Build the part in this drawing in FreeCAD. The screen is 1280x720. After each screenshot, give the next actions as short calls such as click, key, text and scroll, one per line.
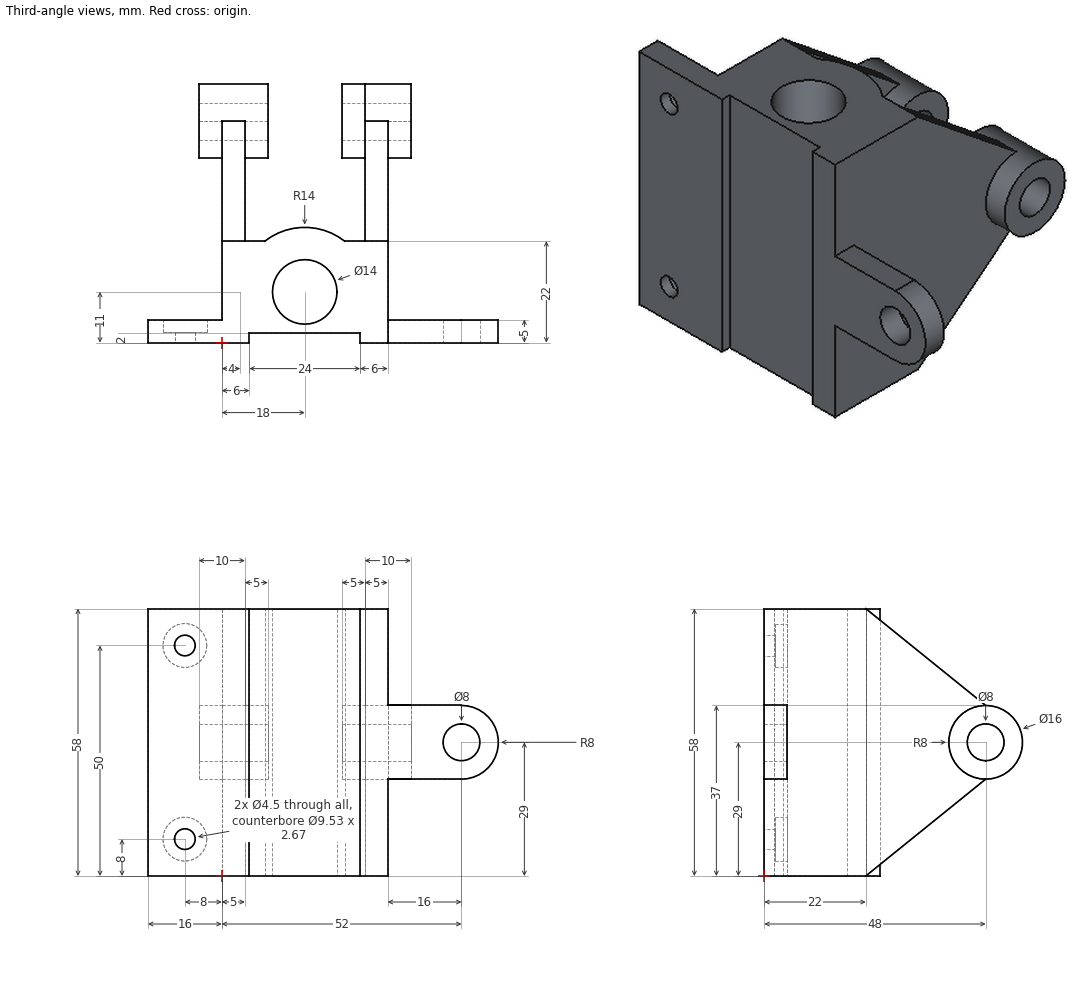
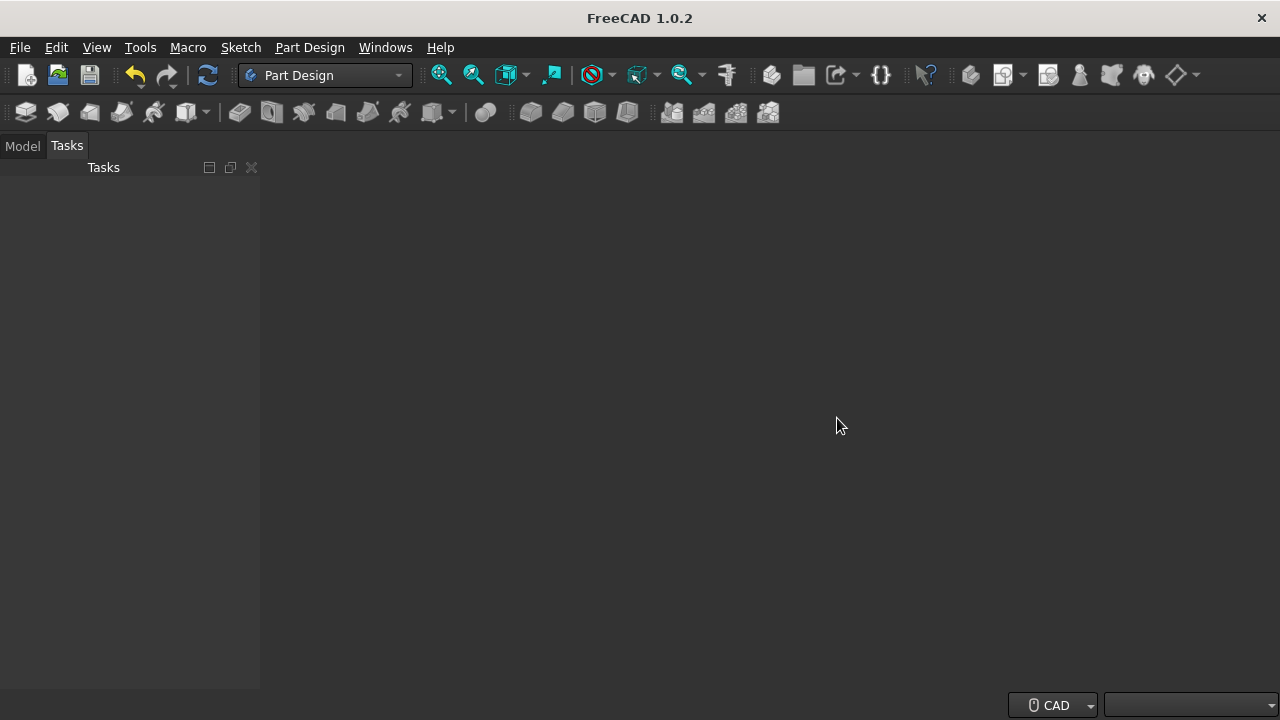
key(ctrl+n)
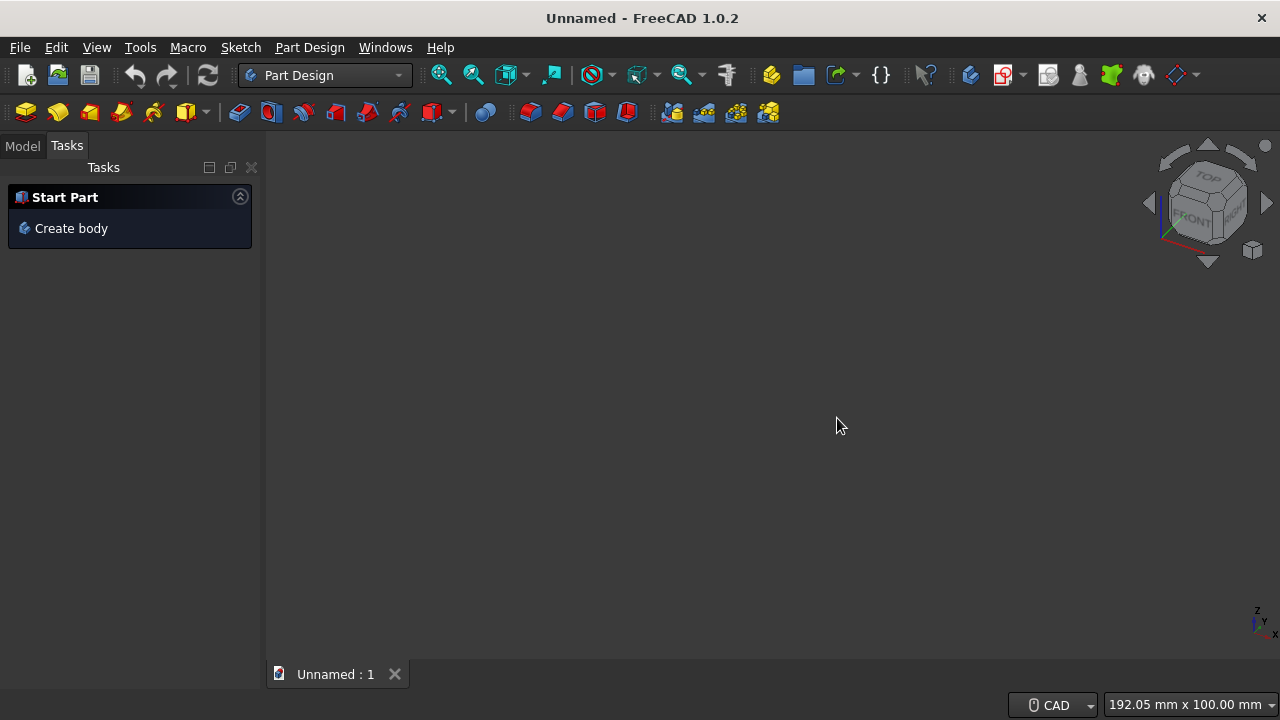
click(1004, 76)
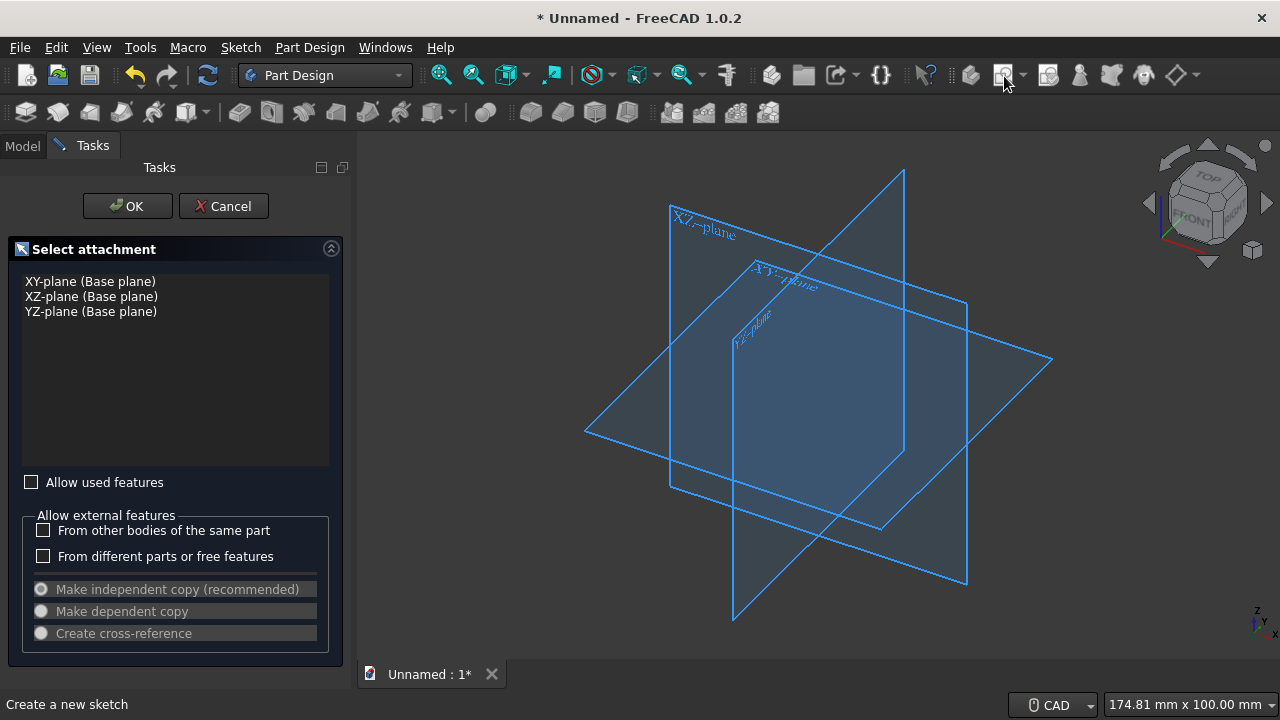
click(82, 282)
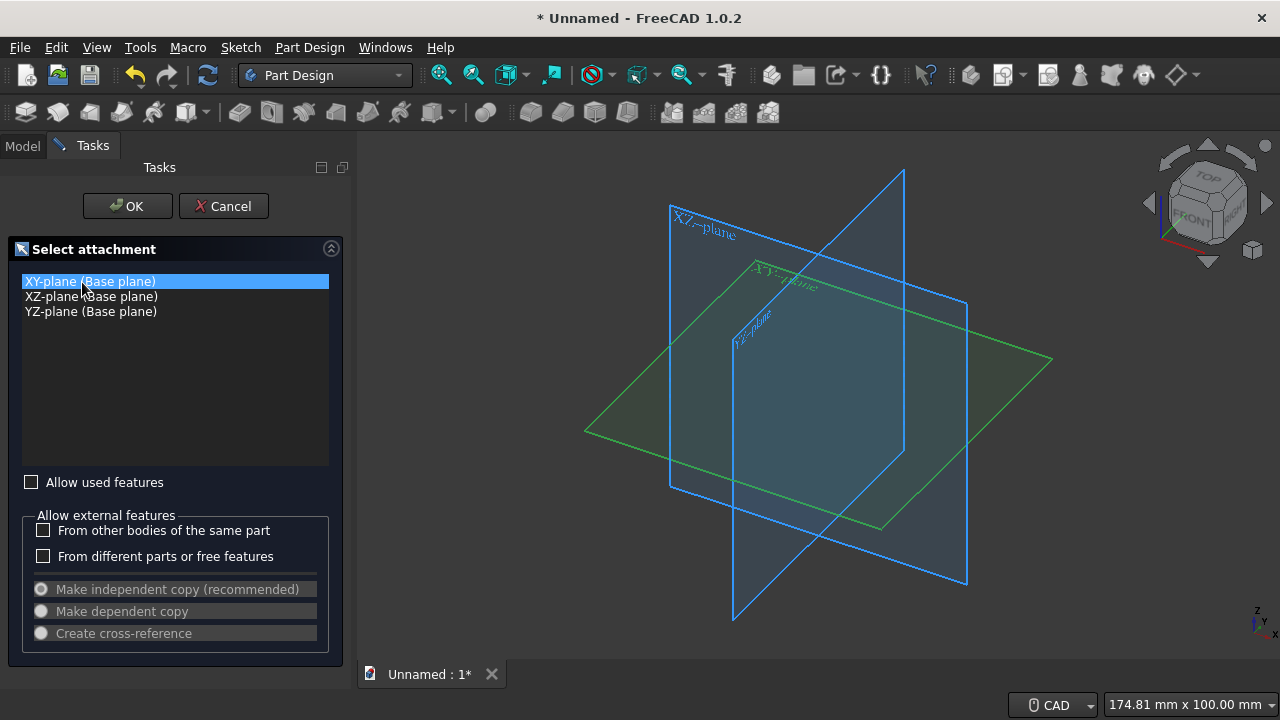
click(128, 206)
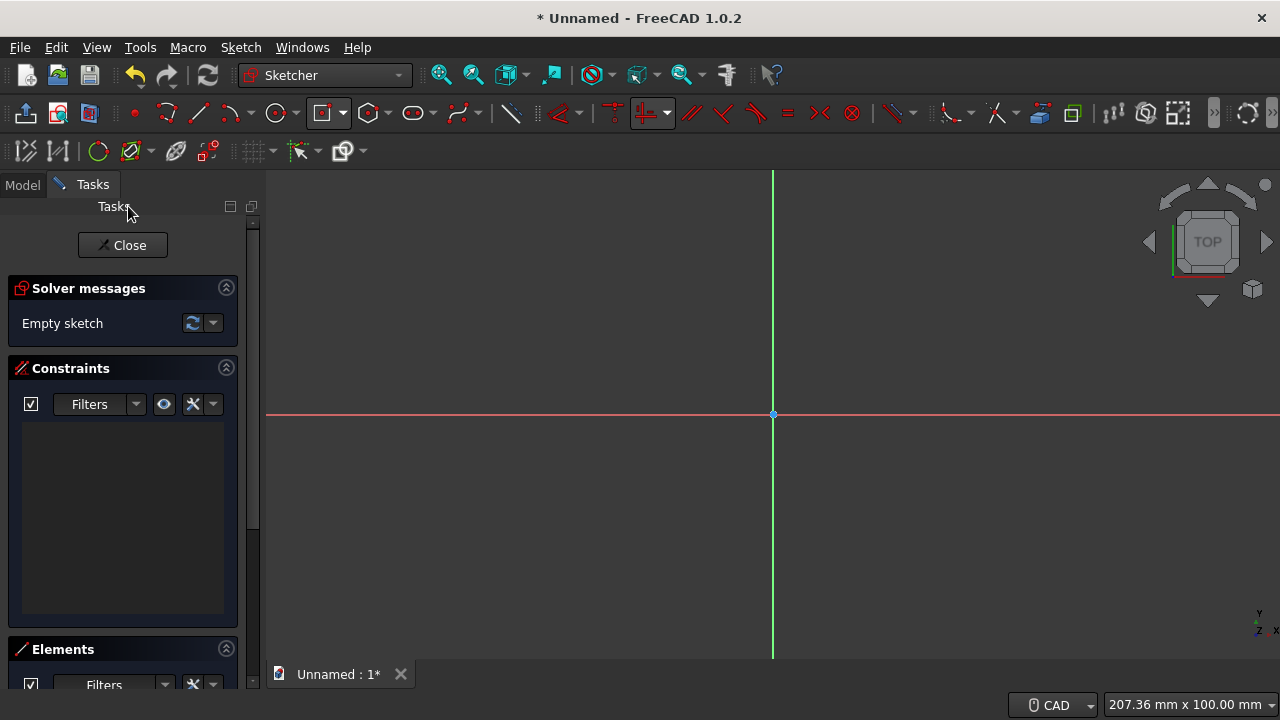
scroll(952, 329, up, 5)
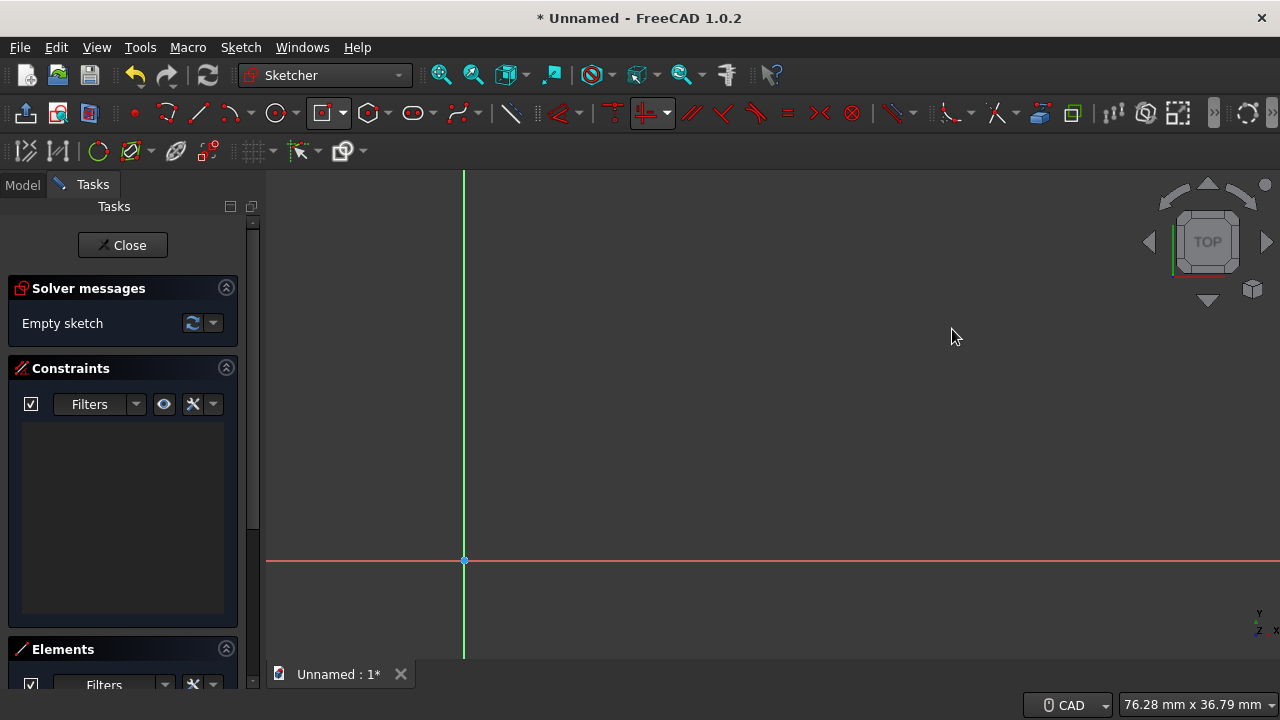
key(g)
key(m)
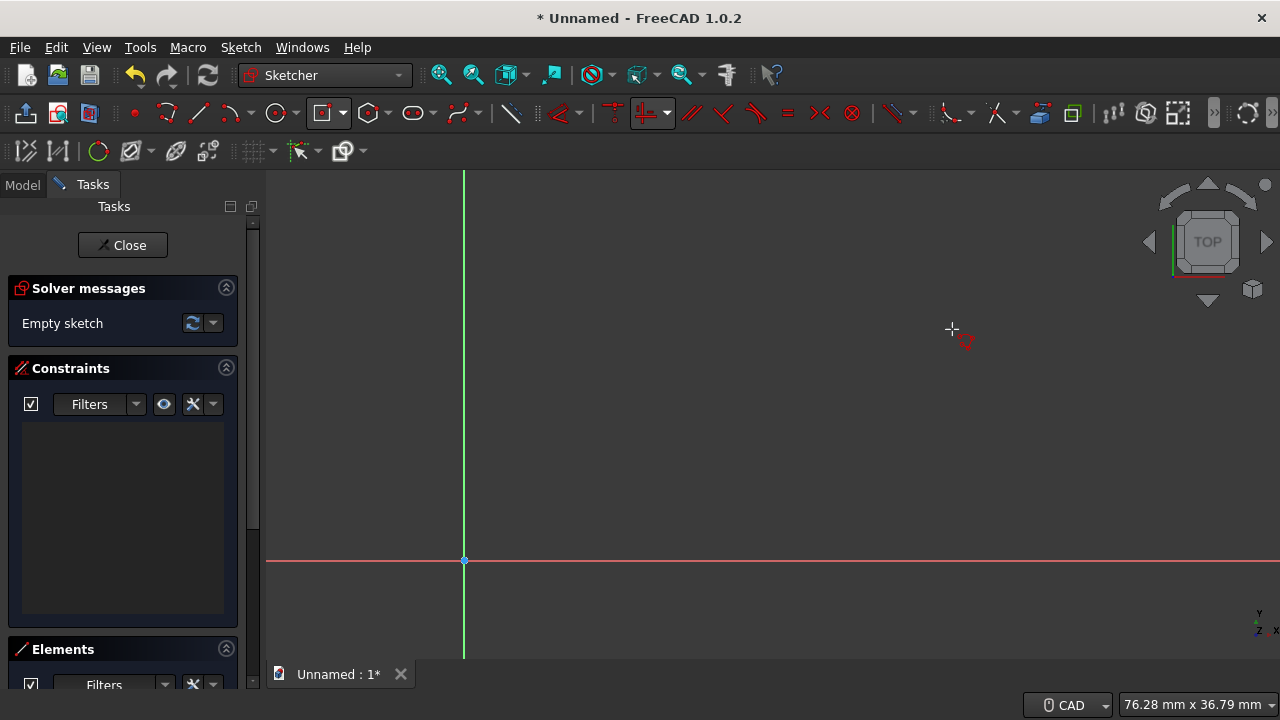
click(464, 561)
click(544, 552)
click(544, 534)
click(863, 534)
click(863, 561)
click(943, 552)
click(943, 268)
click(473, 268)
click(464, 561)
key(Escape)
key(Escape)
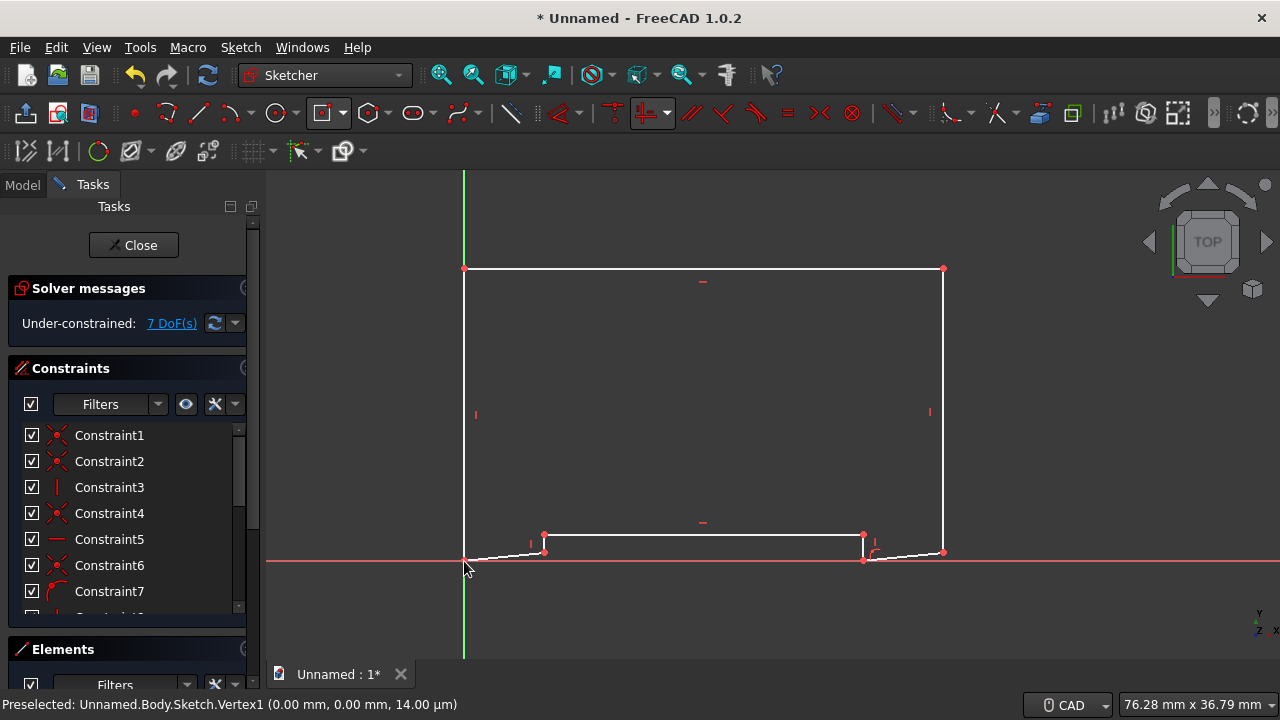
click(488, 558)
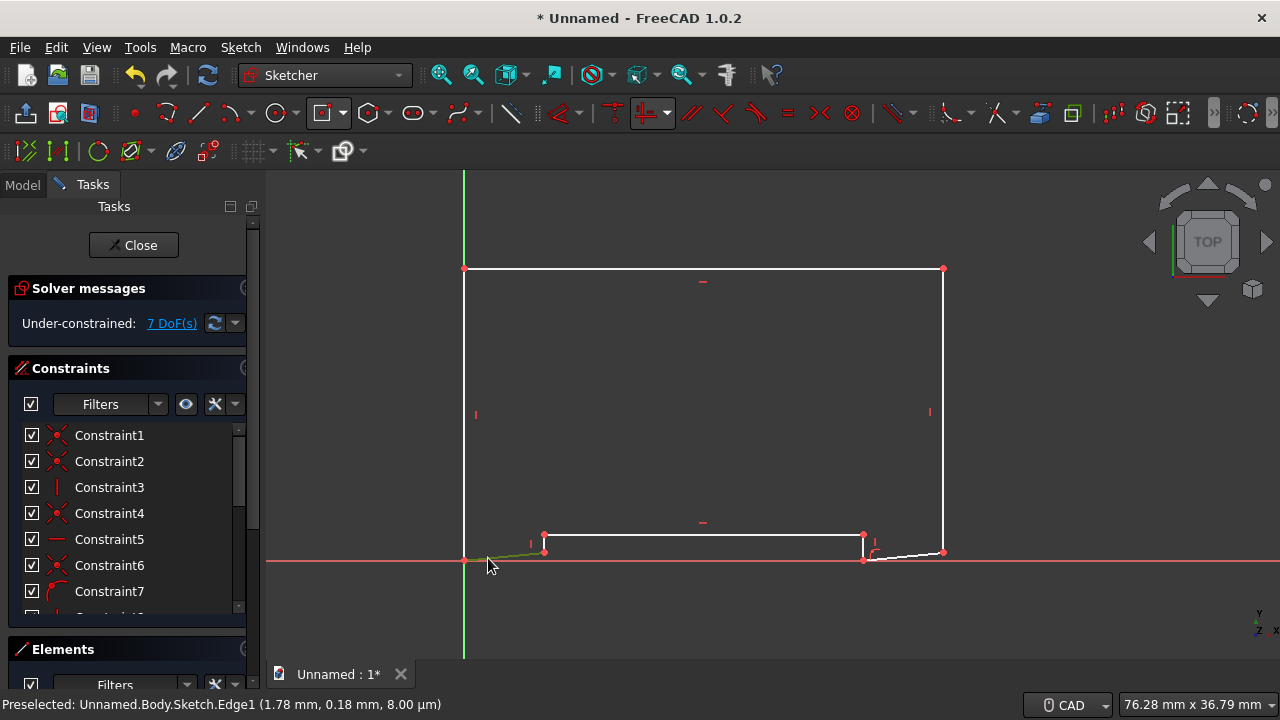
key(h)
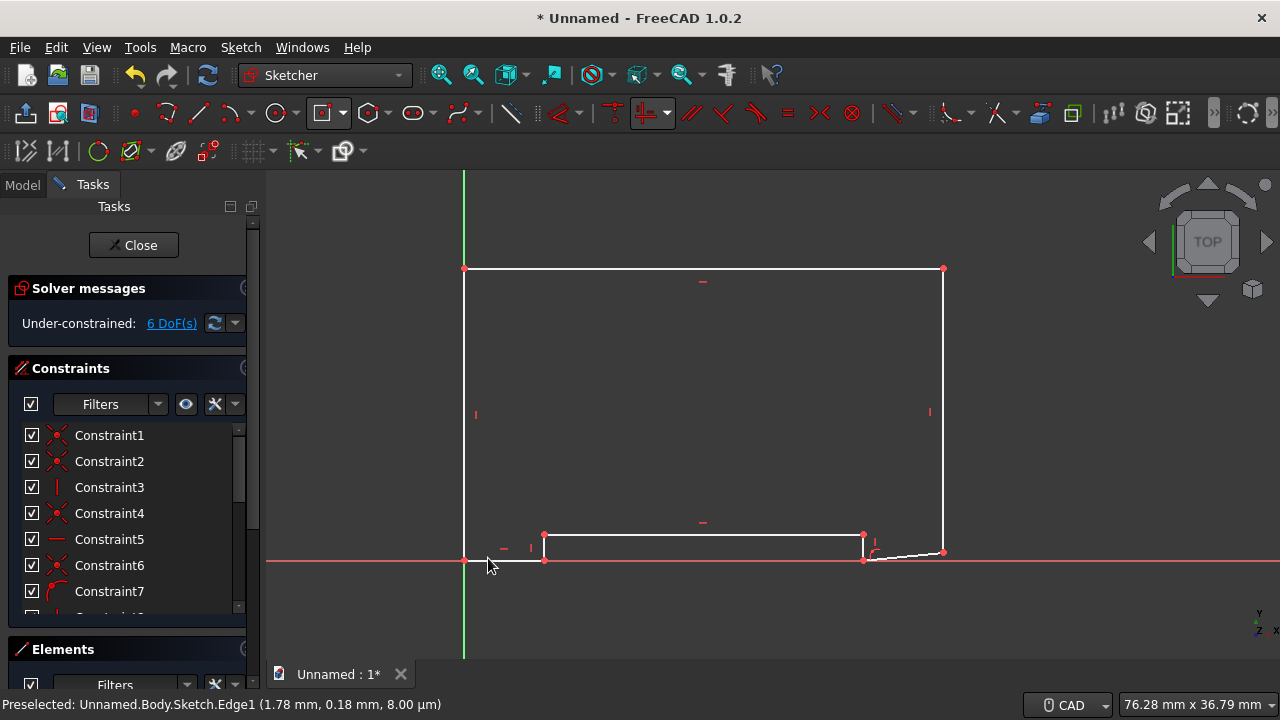
click(887, 558)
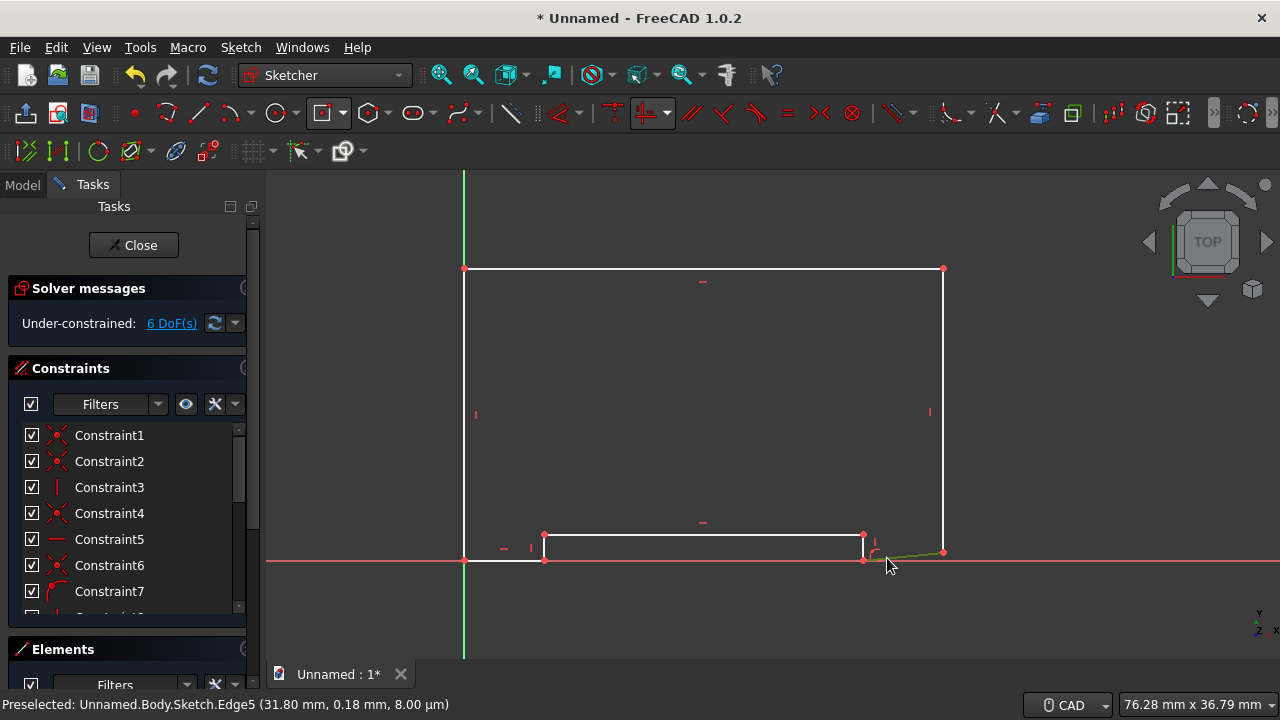
key(h)